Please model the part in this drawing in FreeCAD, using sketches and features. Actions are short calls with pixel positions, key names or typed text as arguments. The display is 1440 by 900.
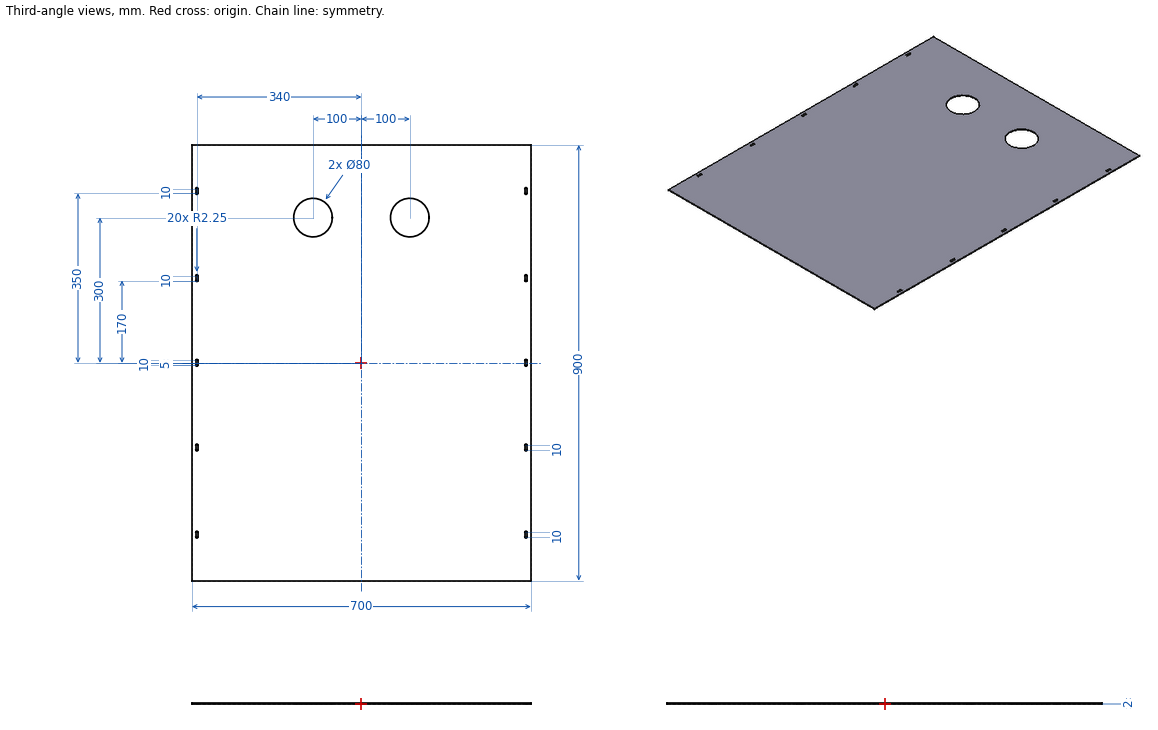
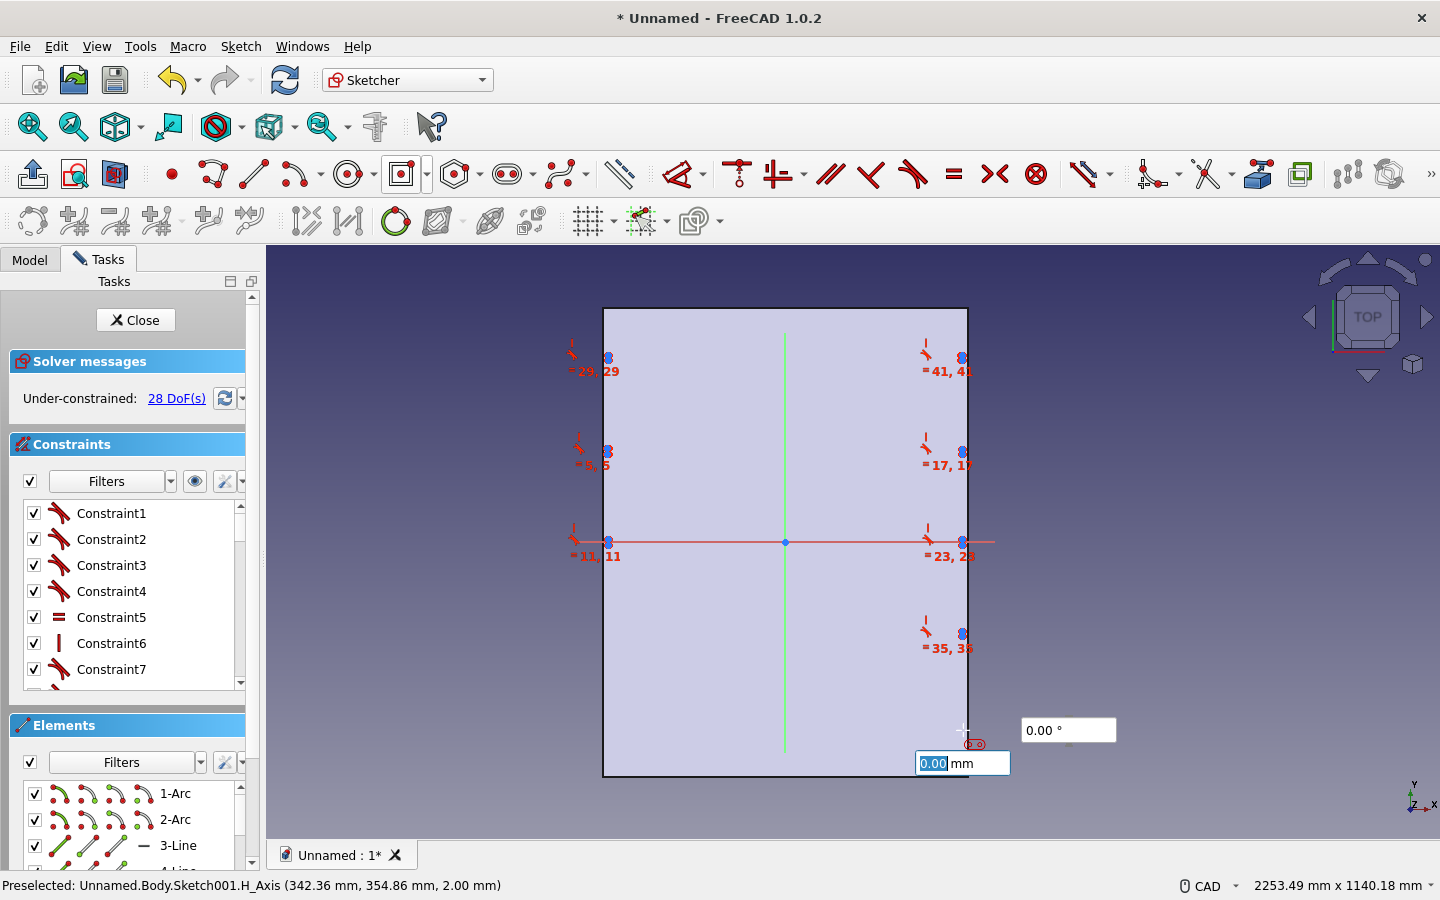
scroll(963, 725, up, 6)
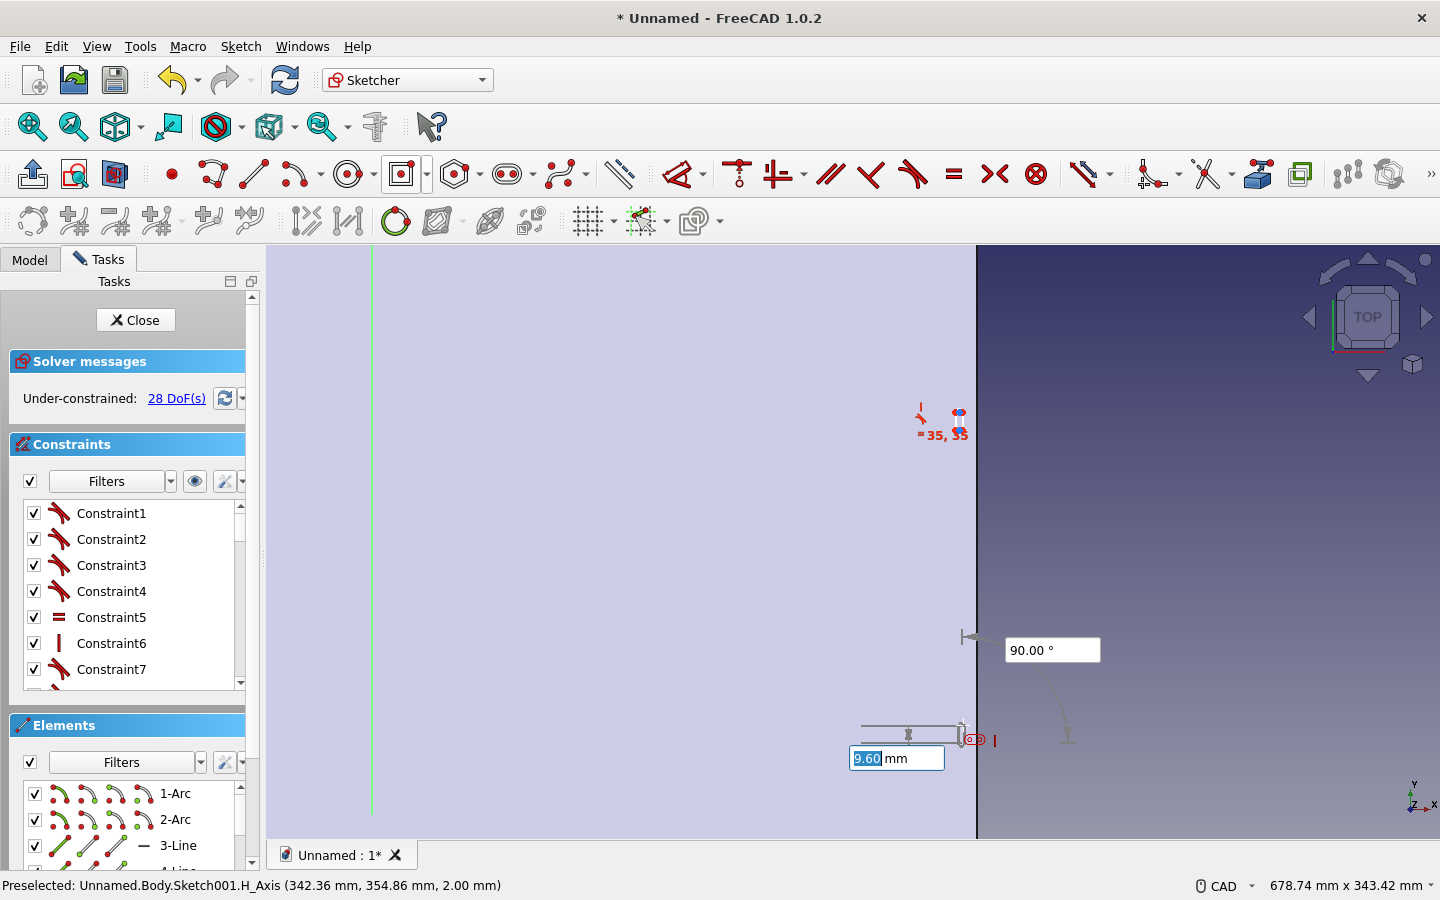
click(962, 722)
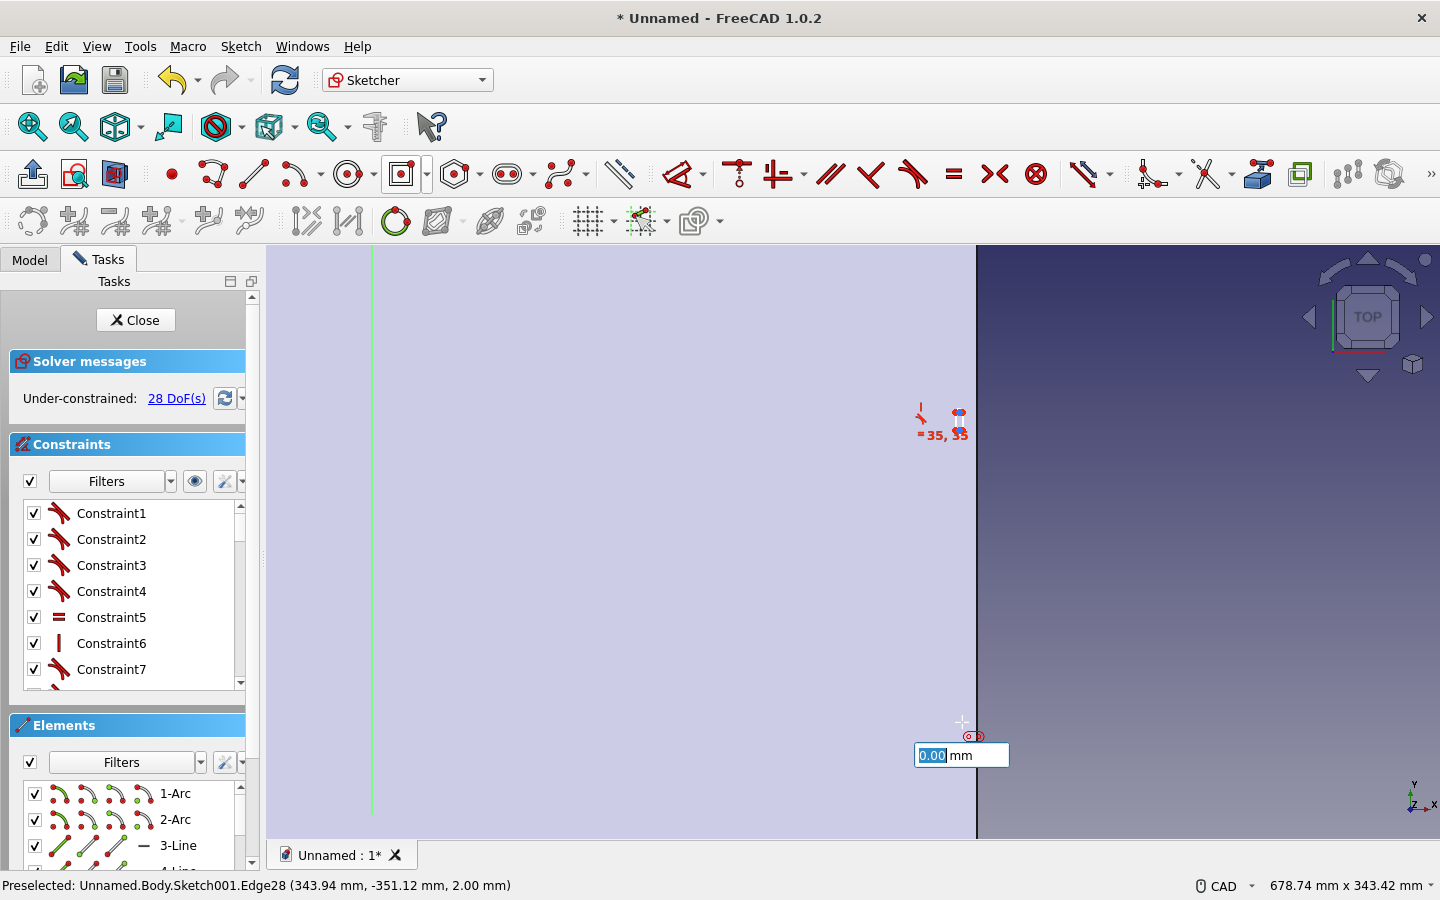
scroll(964, 731, up, 8)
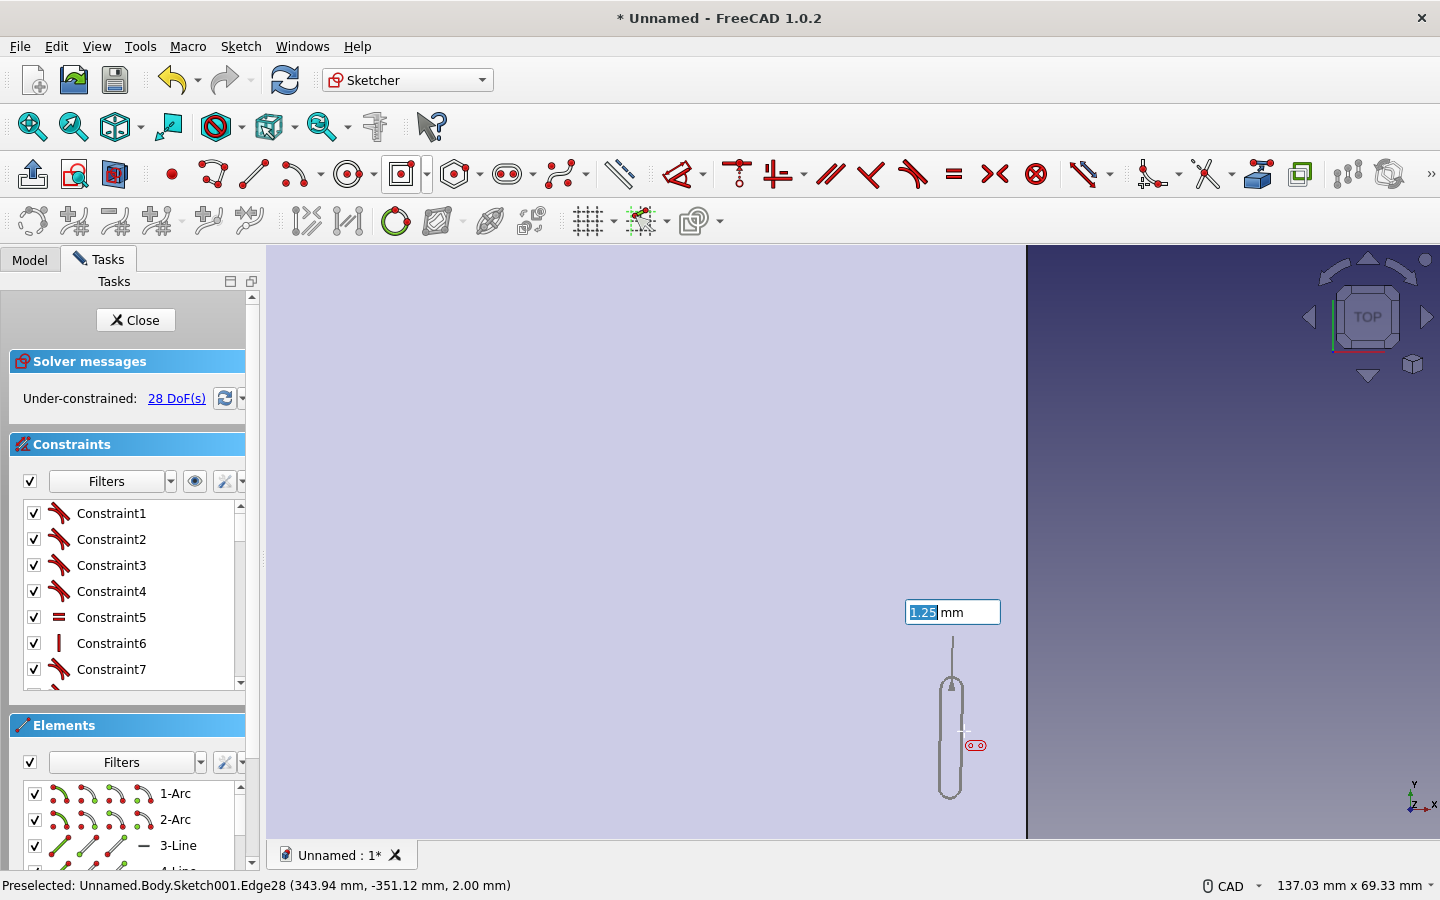
click(961, 727)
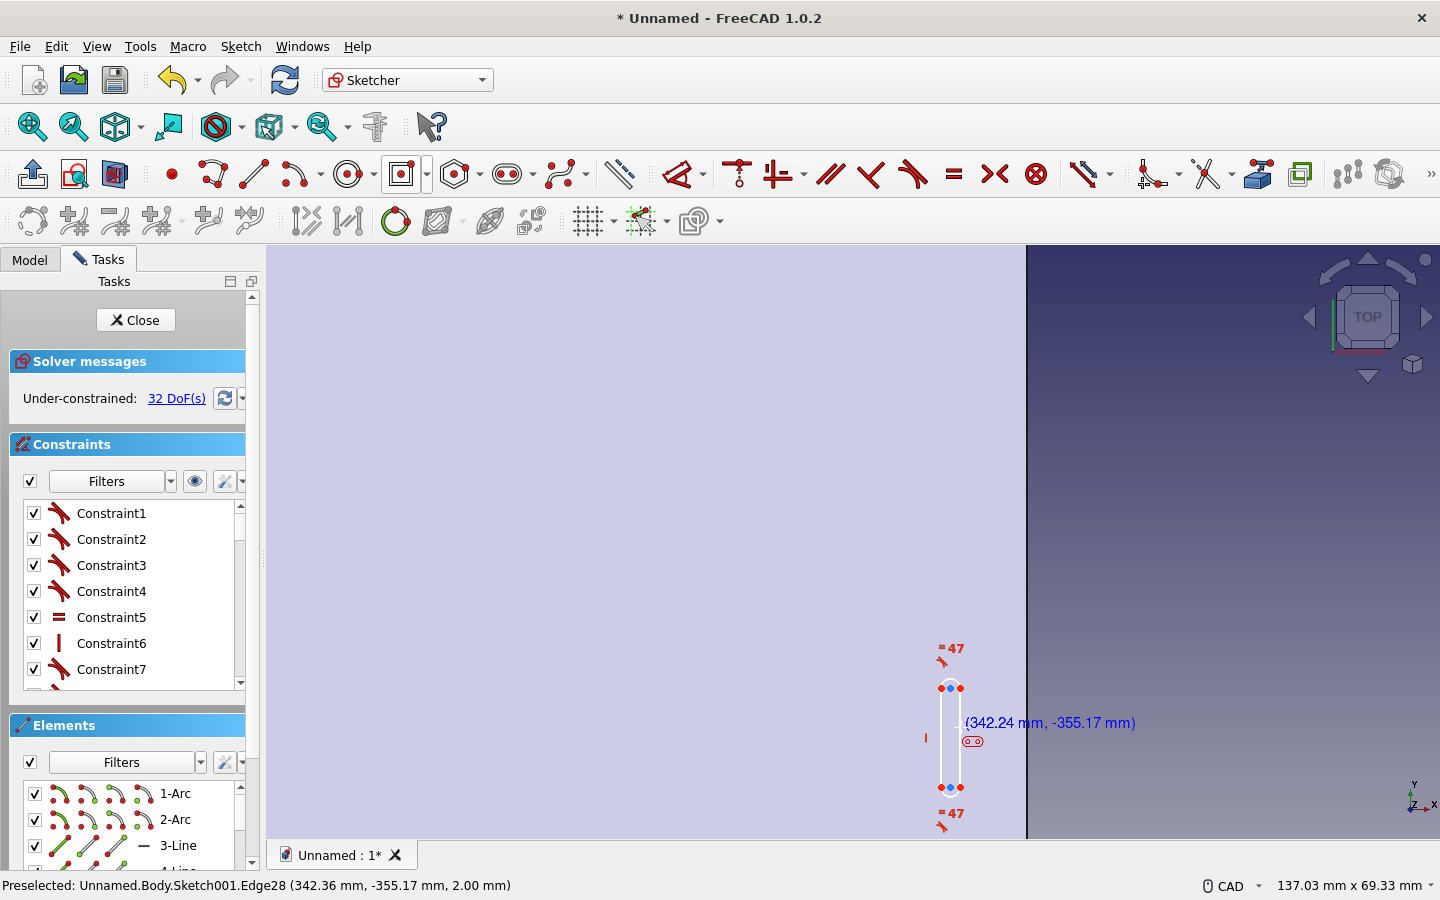
scroll(963, 727, down, 14)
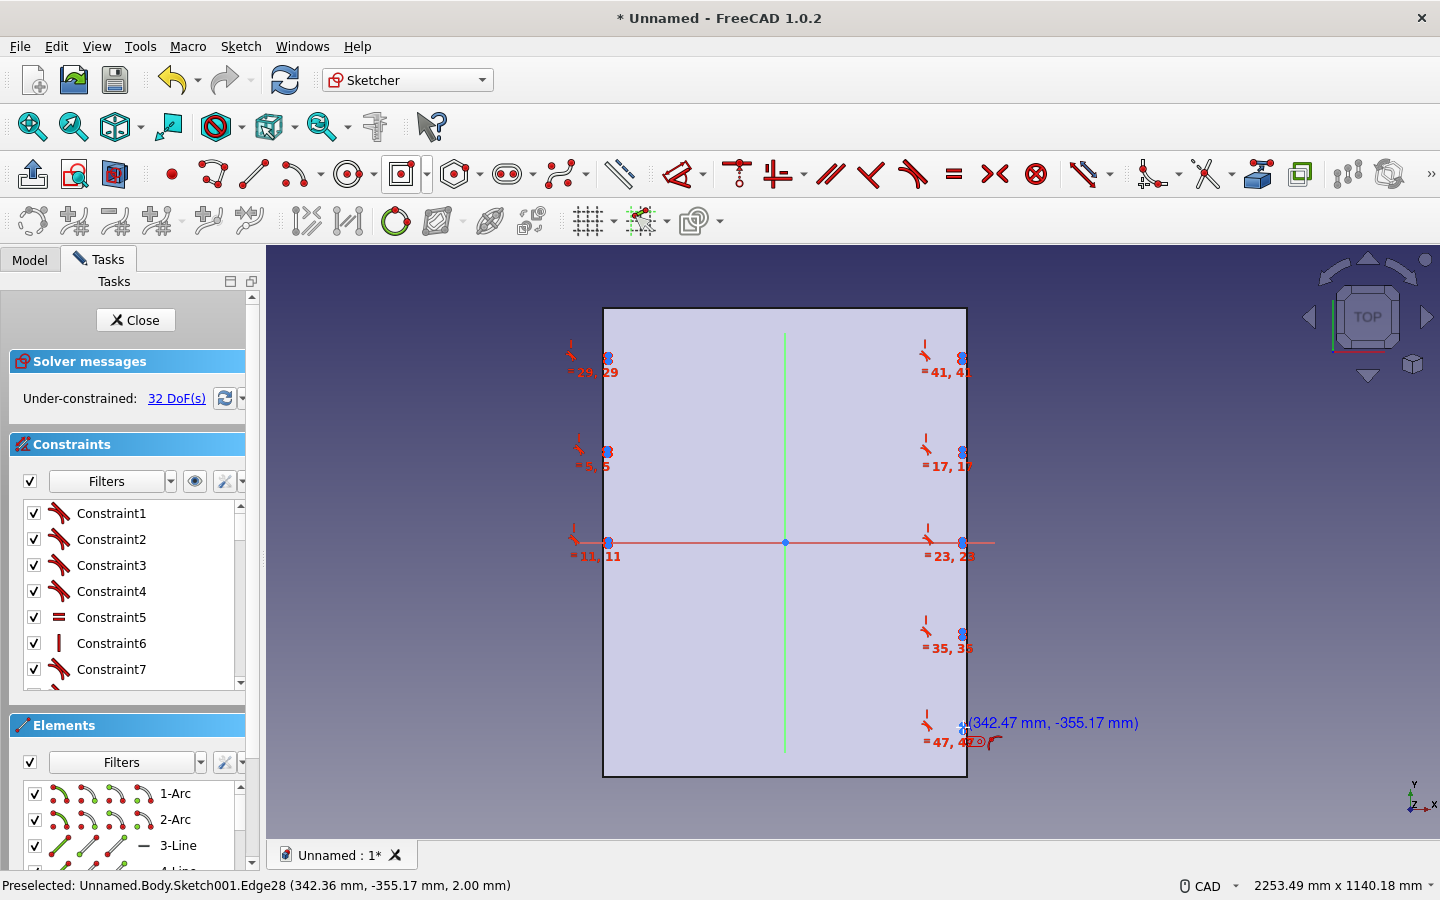
scroll(608, 730, up, 15)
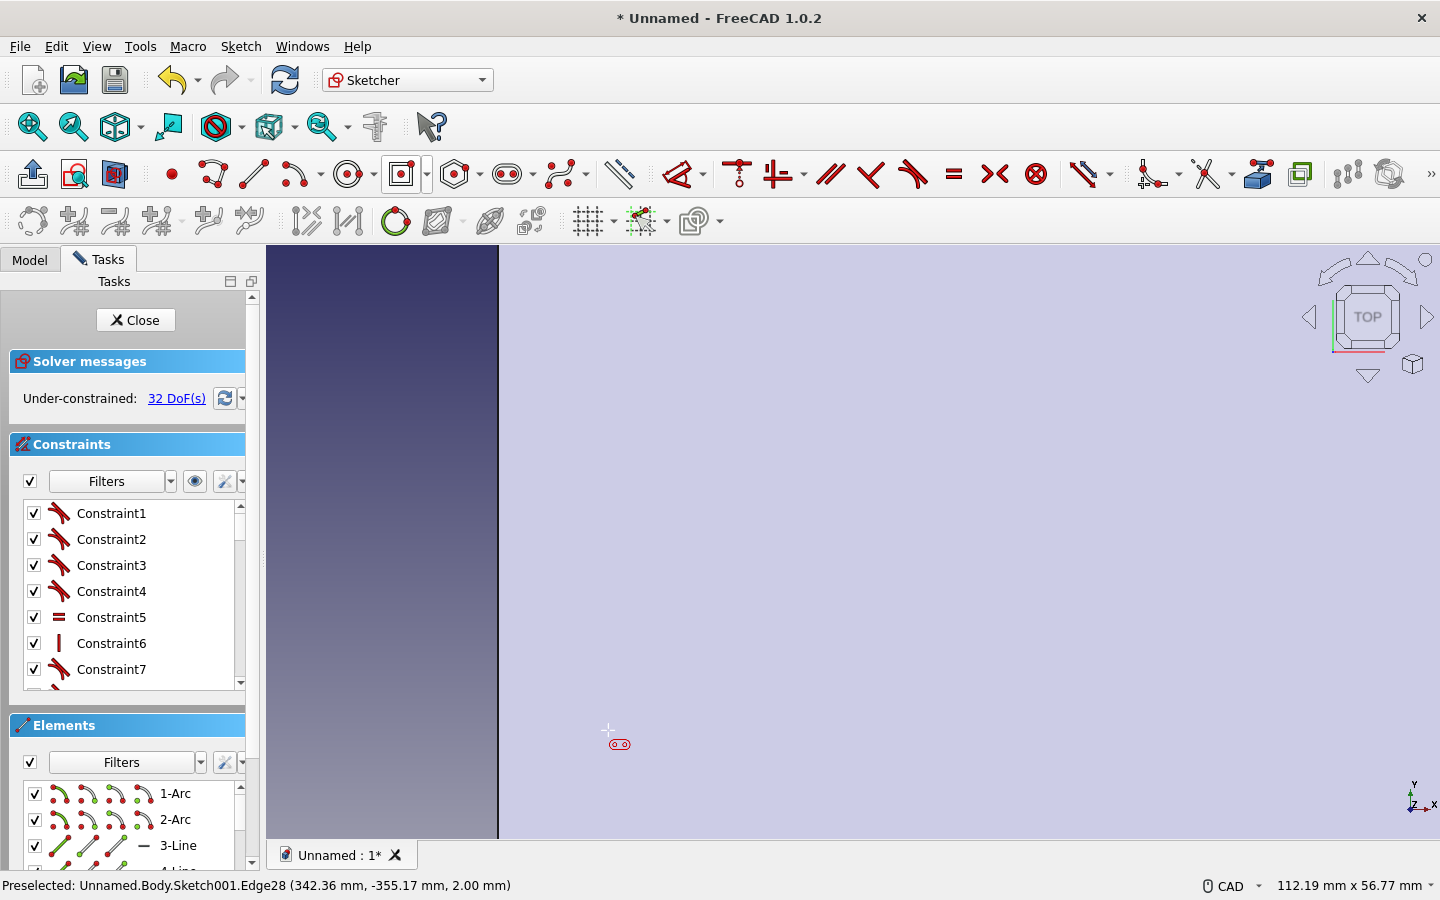
scroll(608, 730, down, 15)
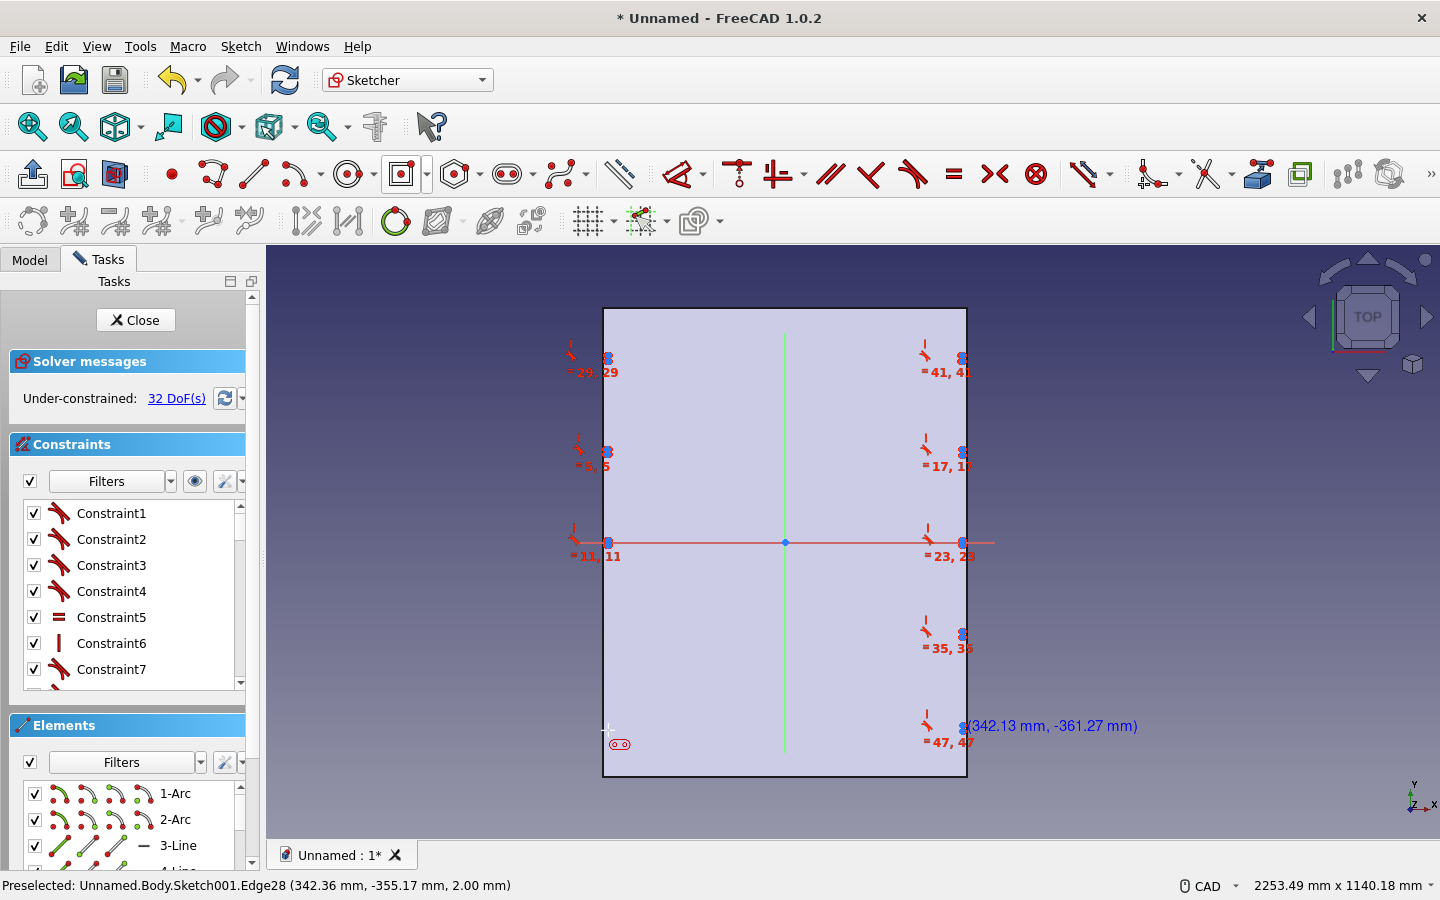
click(608, 730)